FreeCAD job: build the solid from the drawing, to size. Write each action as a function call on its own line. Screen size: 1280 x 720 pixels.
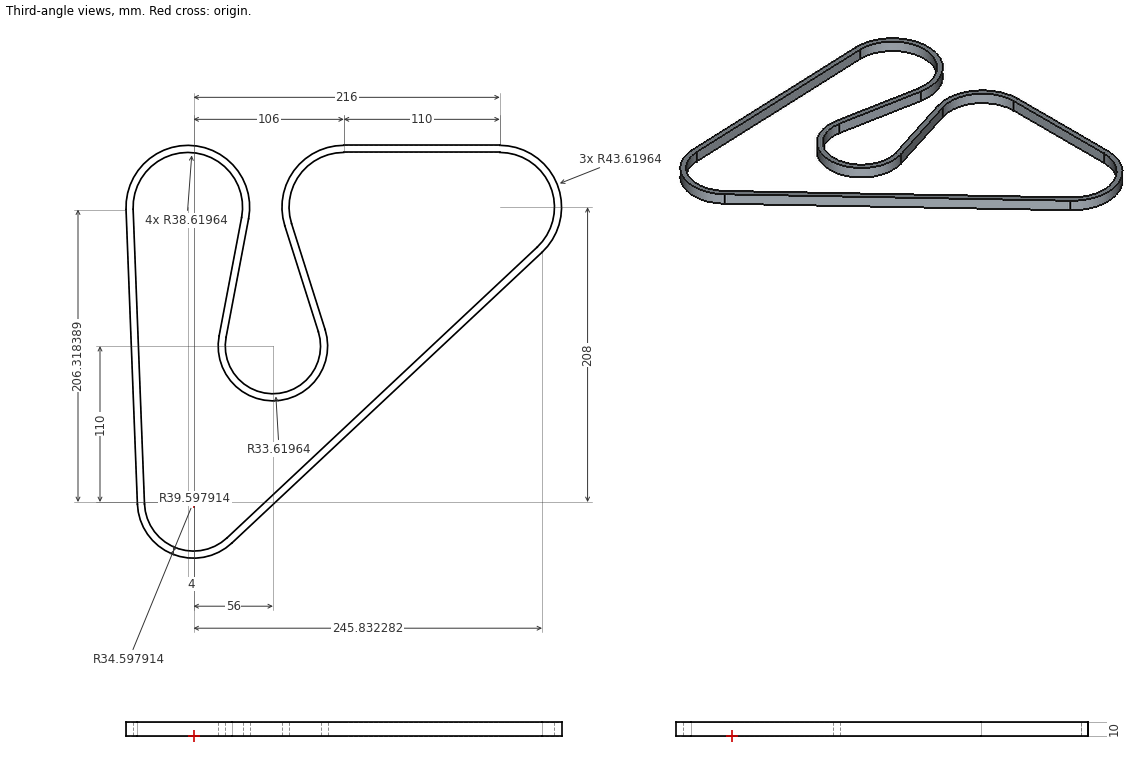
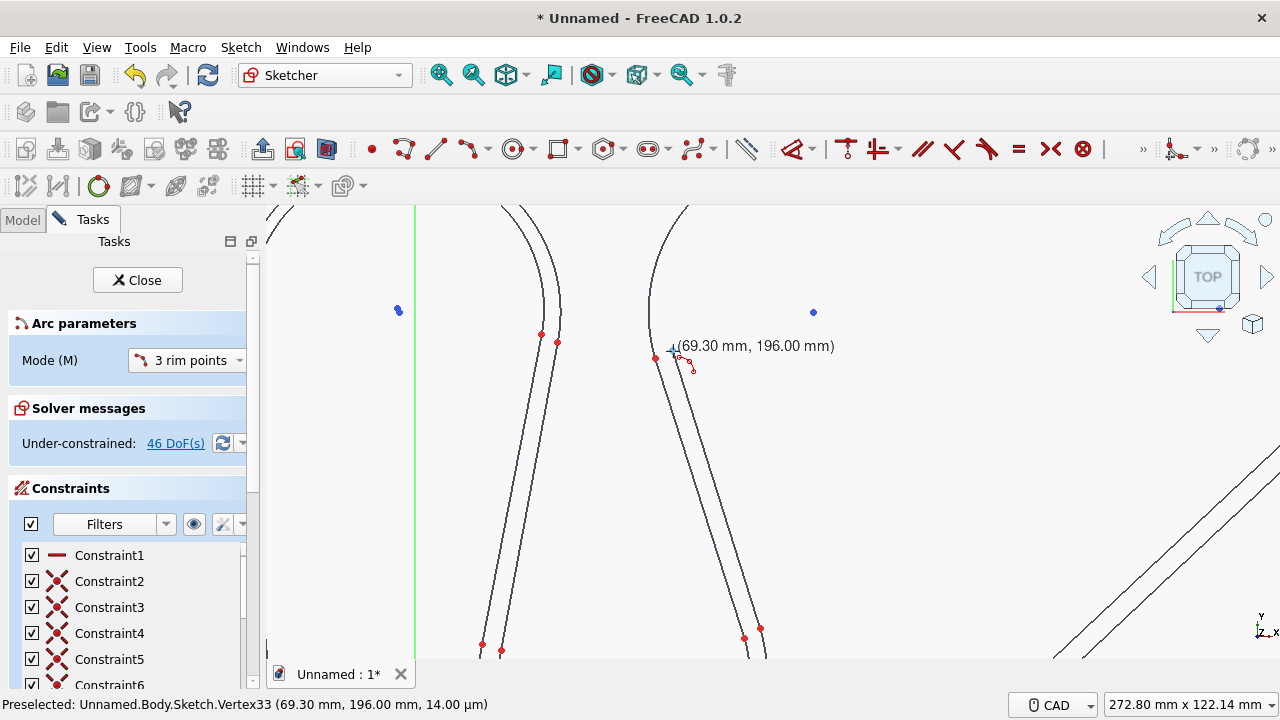
scroll(672, 351, down, 7)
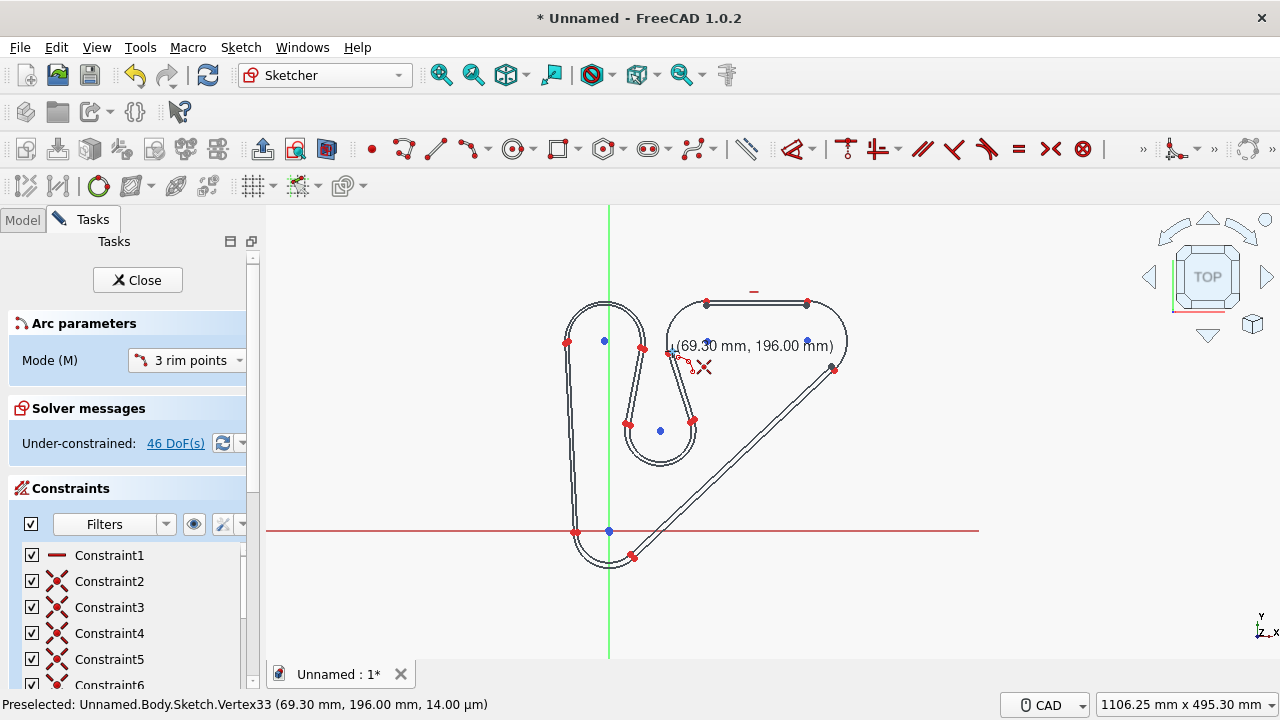
scroll(706, 305, up, 7)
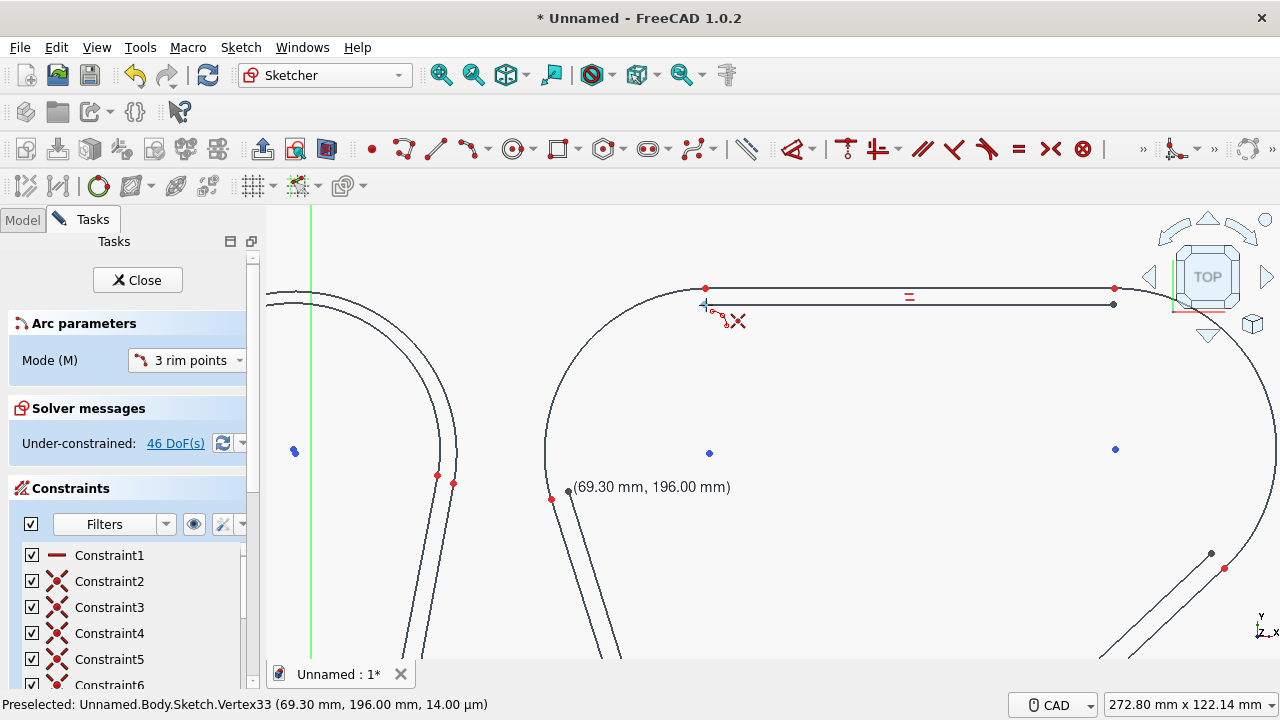
click(705, 305)
click(576, 385)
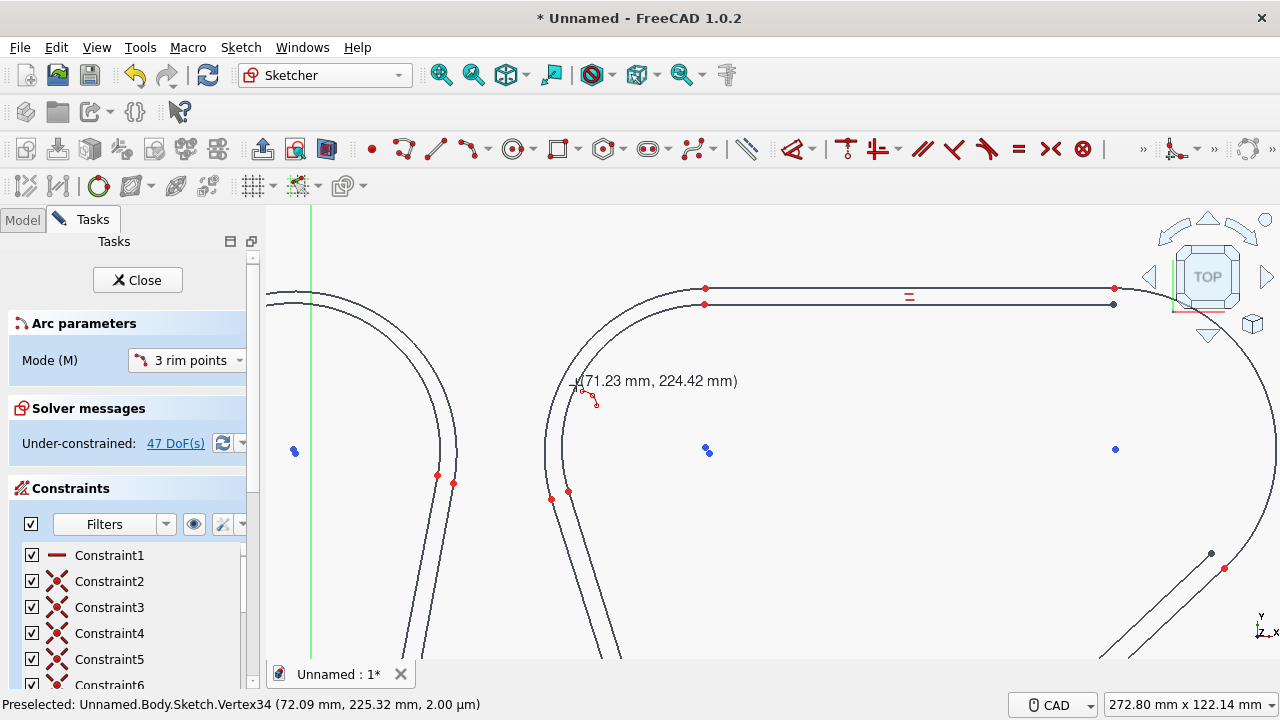
click(1114, 305)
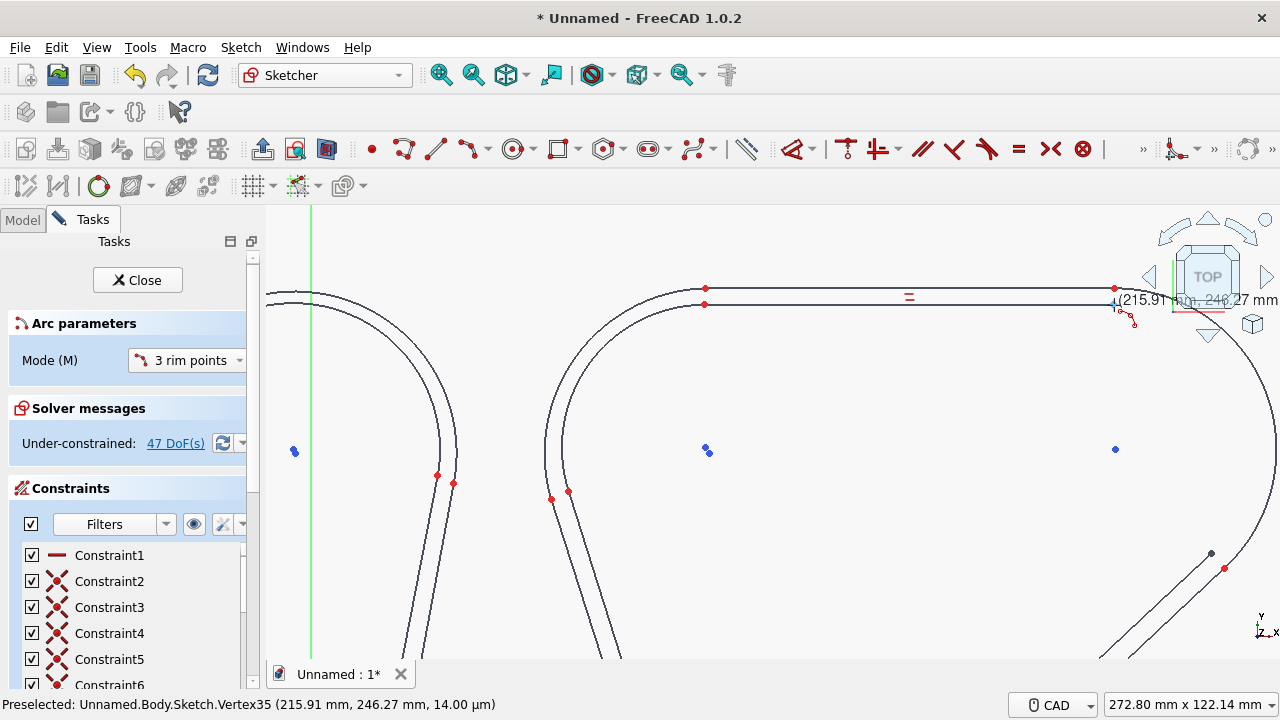
scroll(706, 305, down, 7)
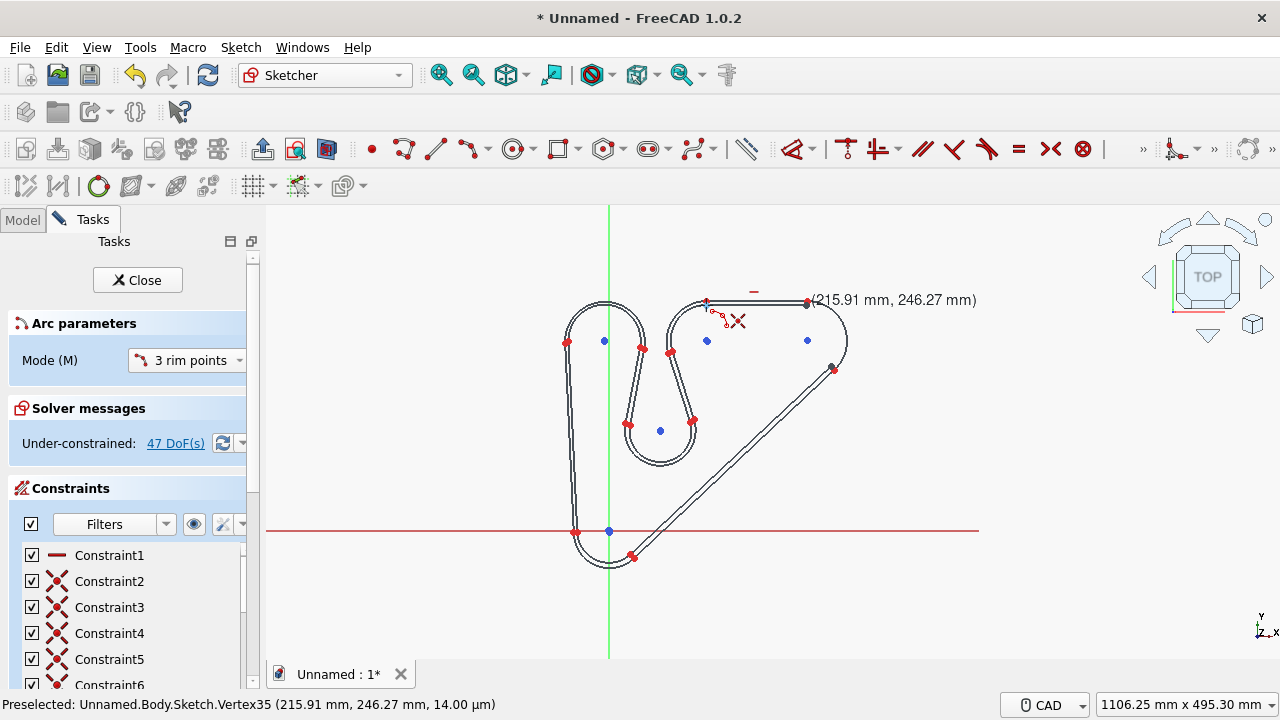
scroll(831, 366, up, 7)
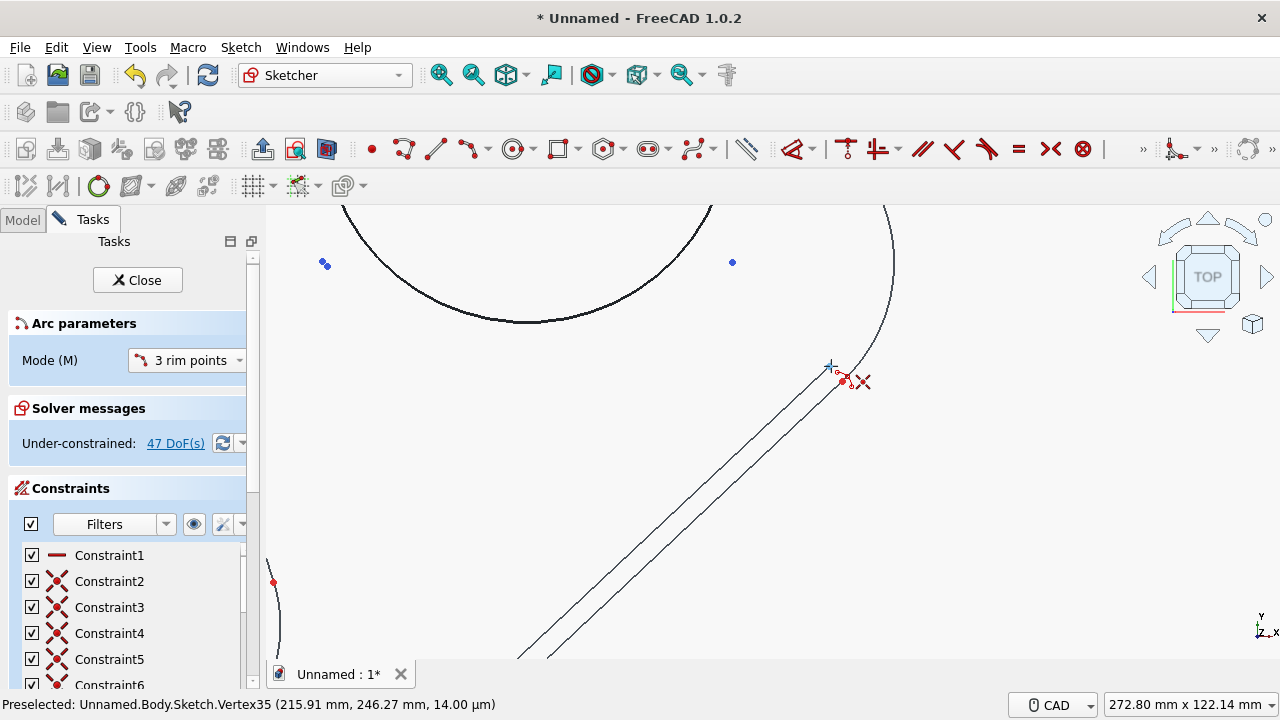
click(830, 366)
click(875, 275)
key(Escape)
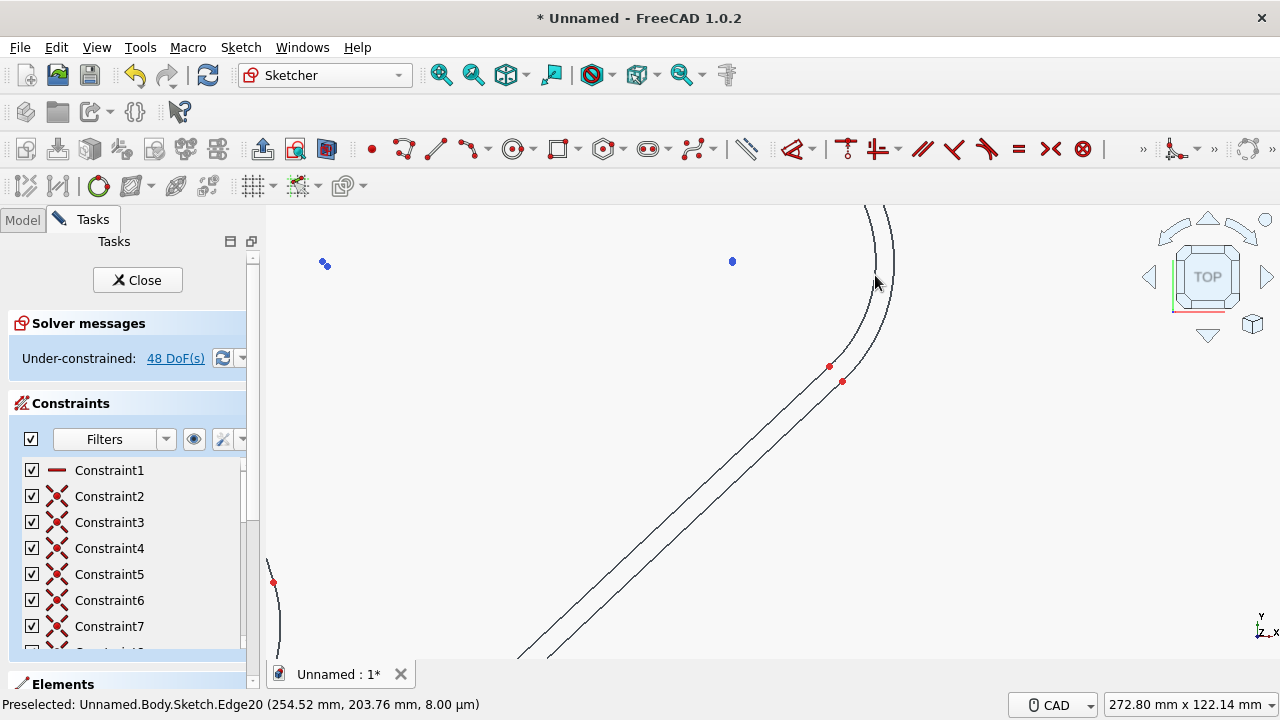
click(599, 610)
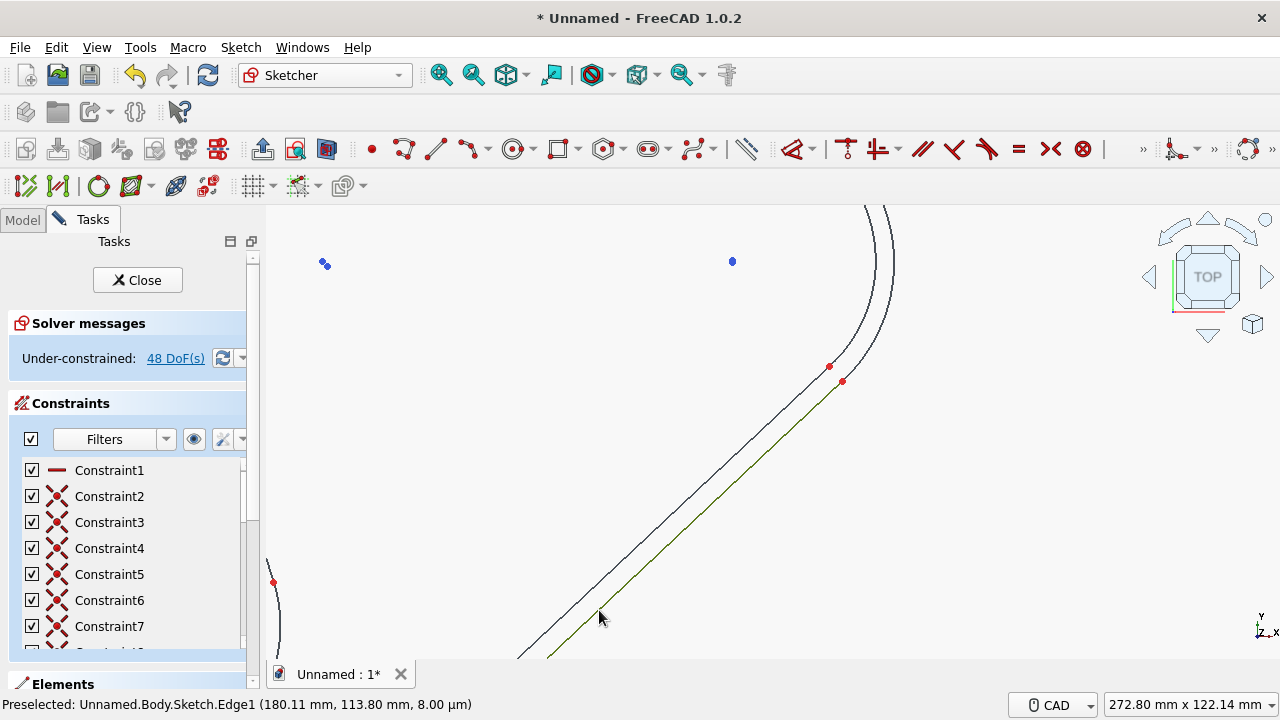
scroll(831, 366, down, 7)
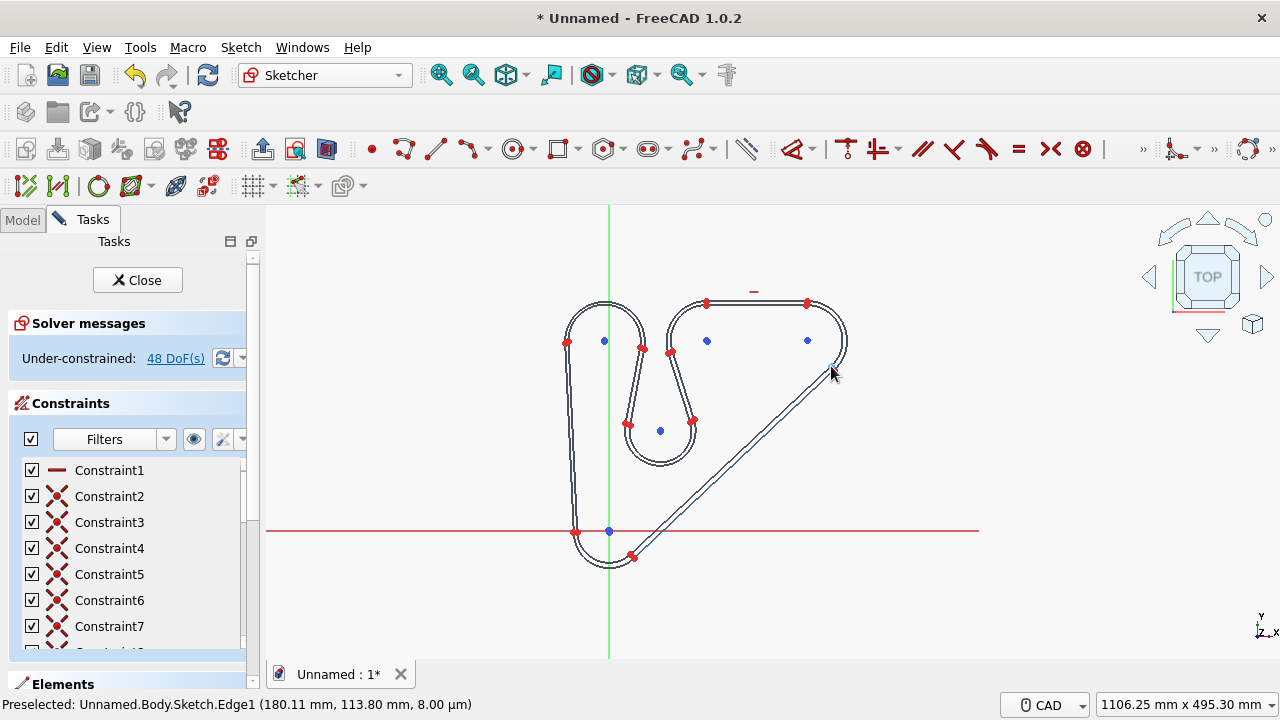
scroll(582, 555, up, 6)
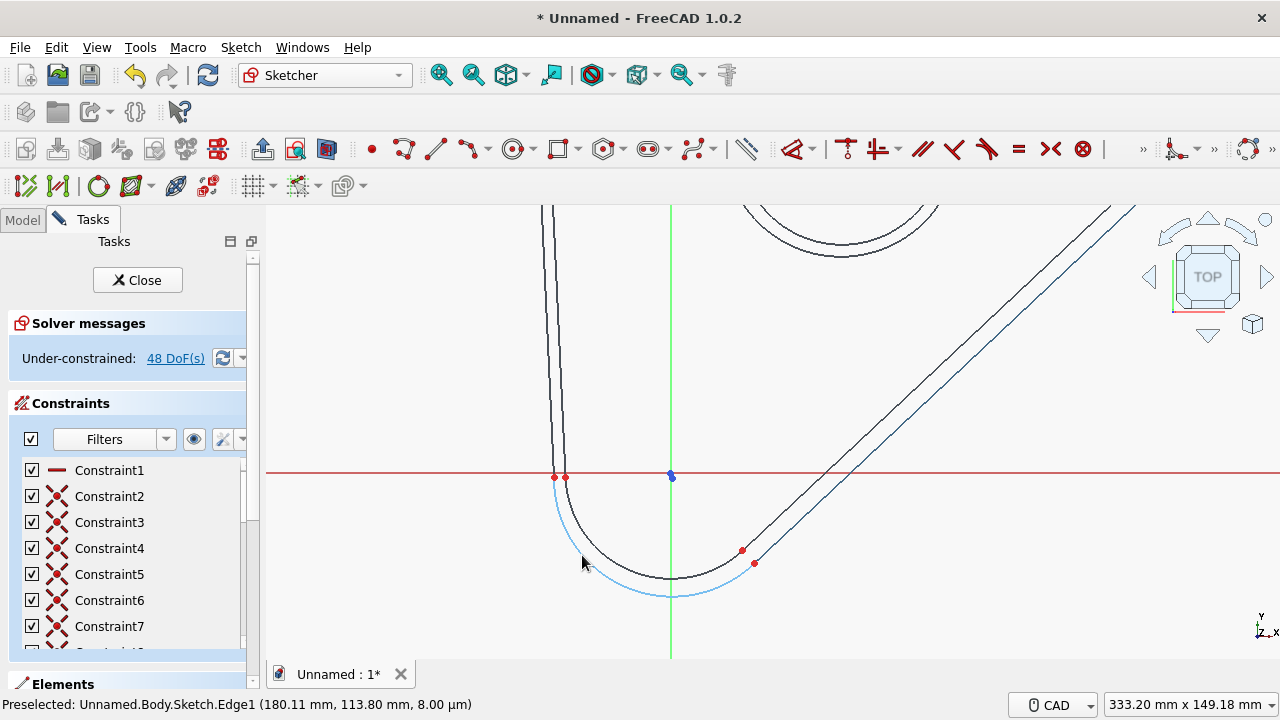
click(582, 554)